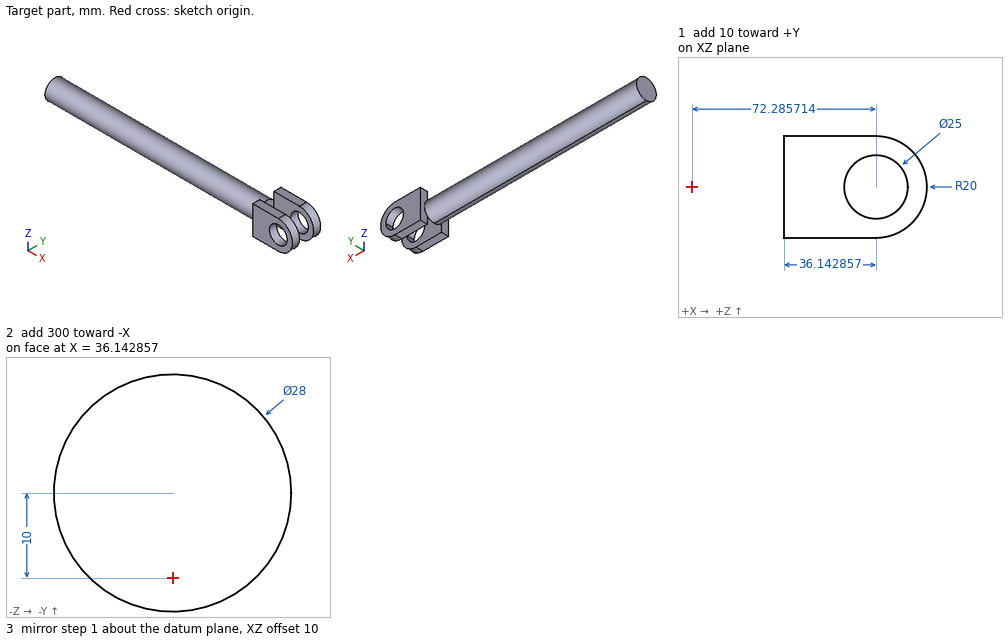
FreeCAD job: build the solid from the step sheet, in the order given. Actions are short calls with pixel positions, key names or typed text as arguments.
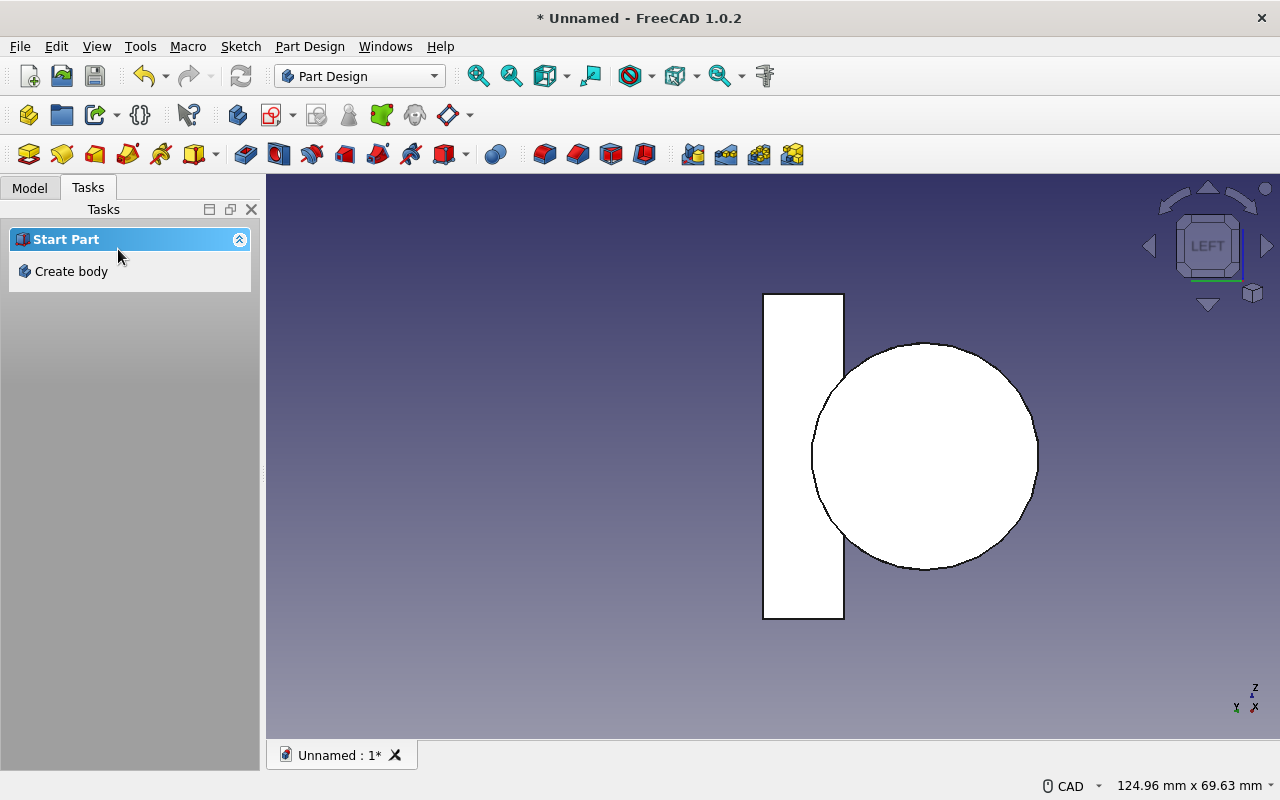
click(30, 188)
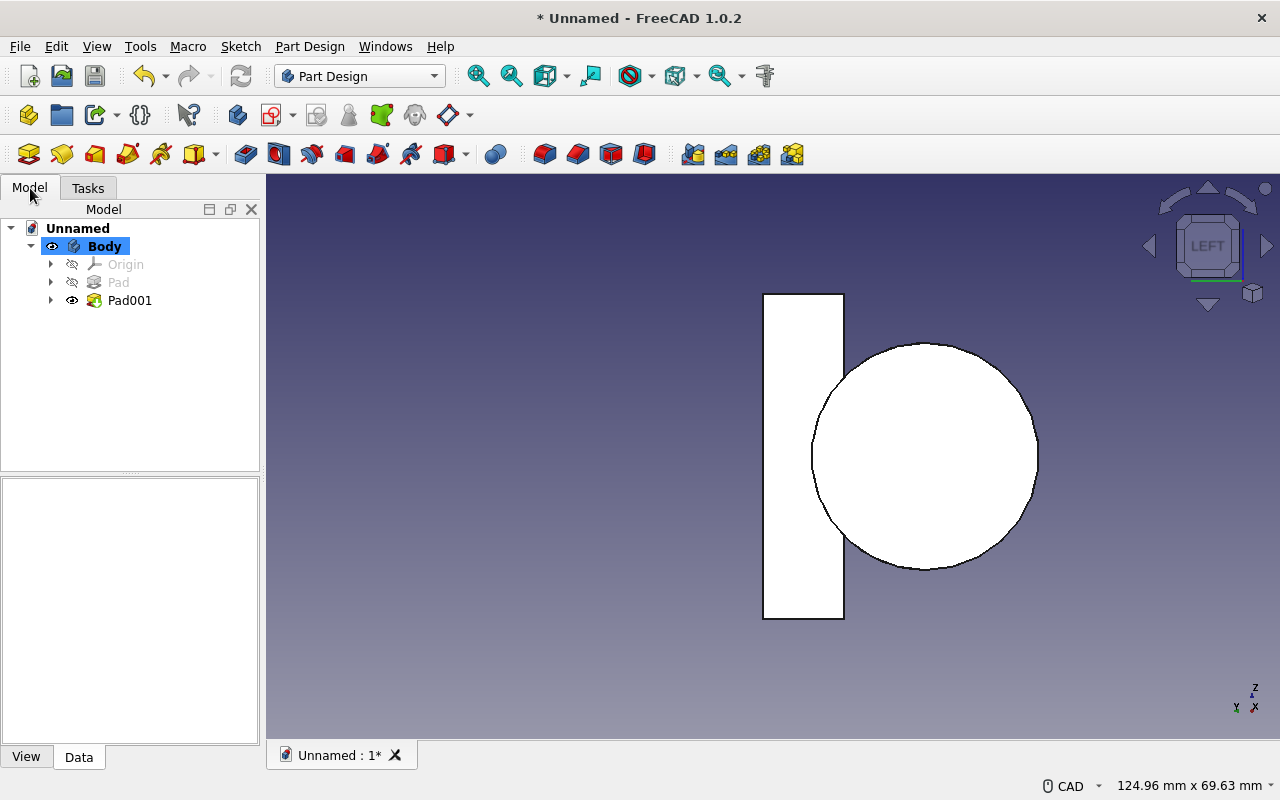
click(51, 264)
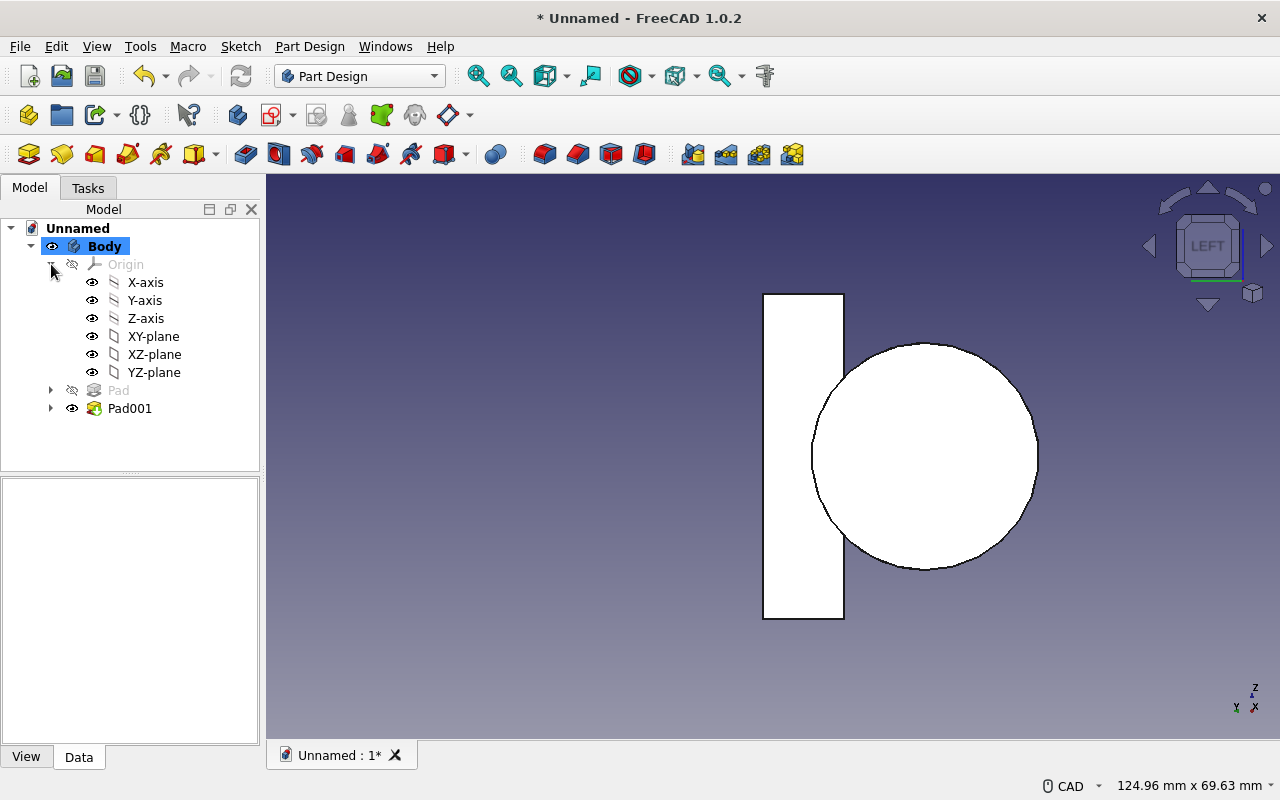
click(137, 354)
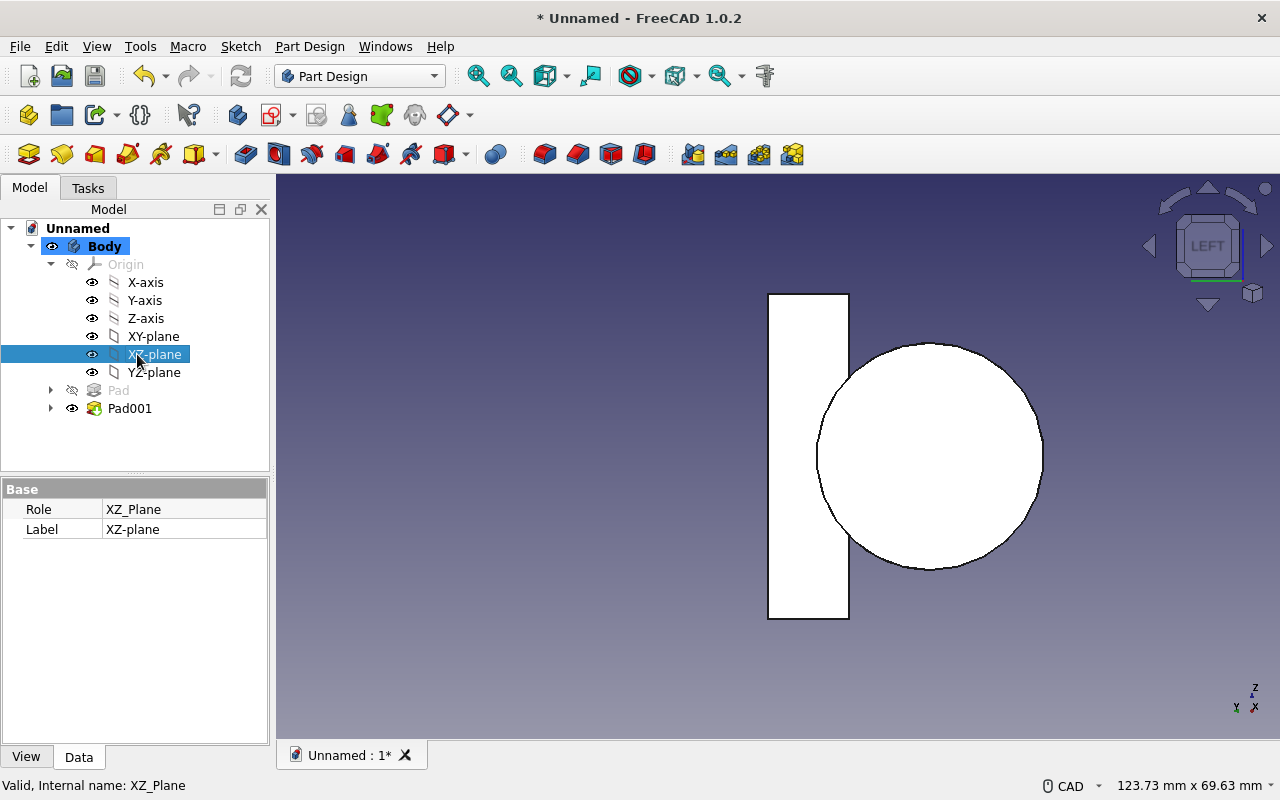
click(448, 116)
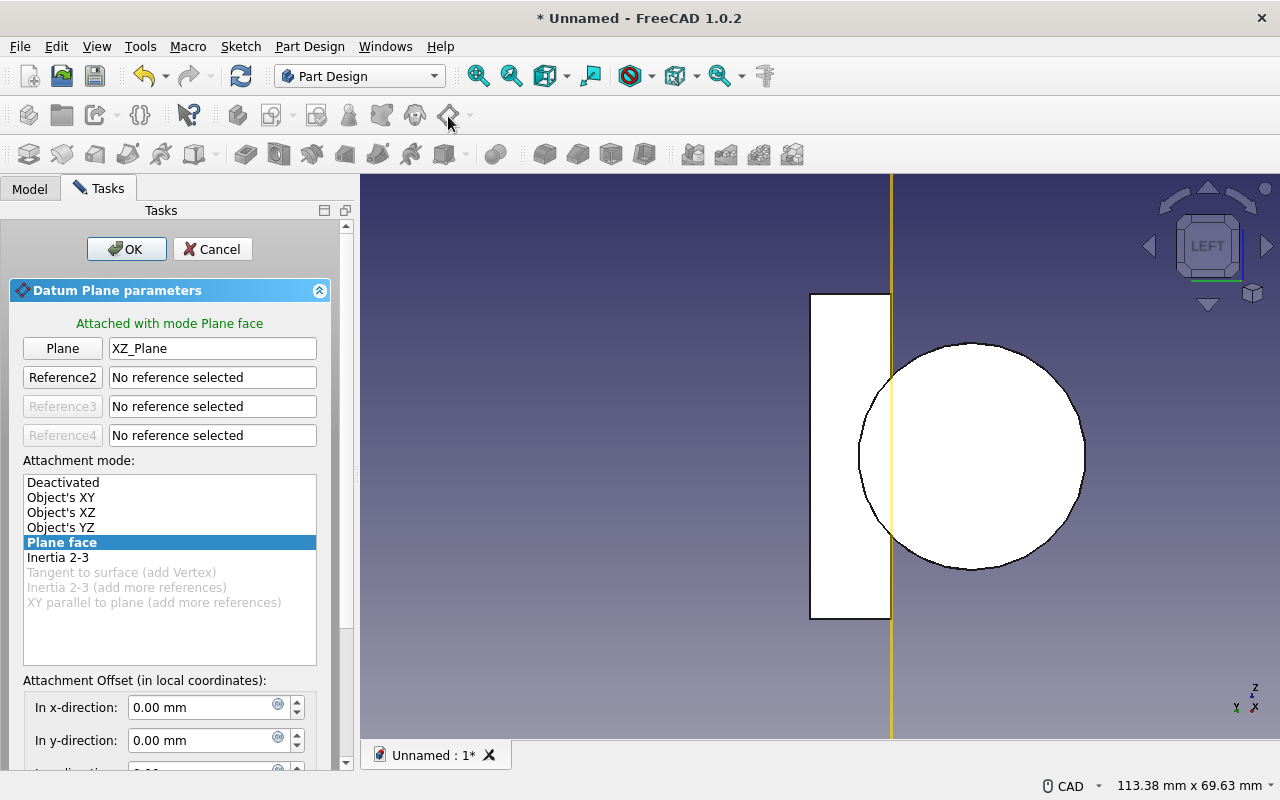
scroll(346, 495, down, 2)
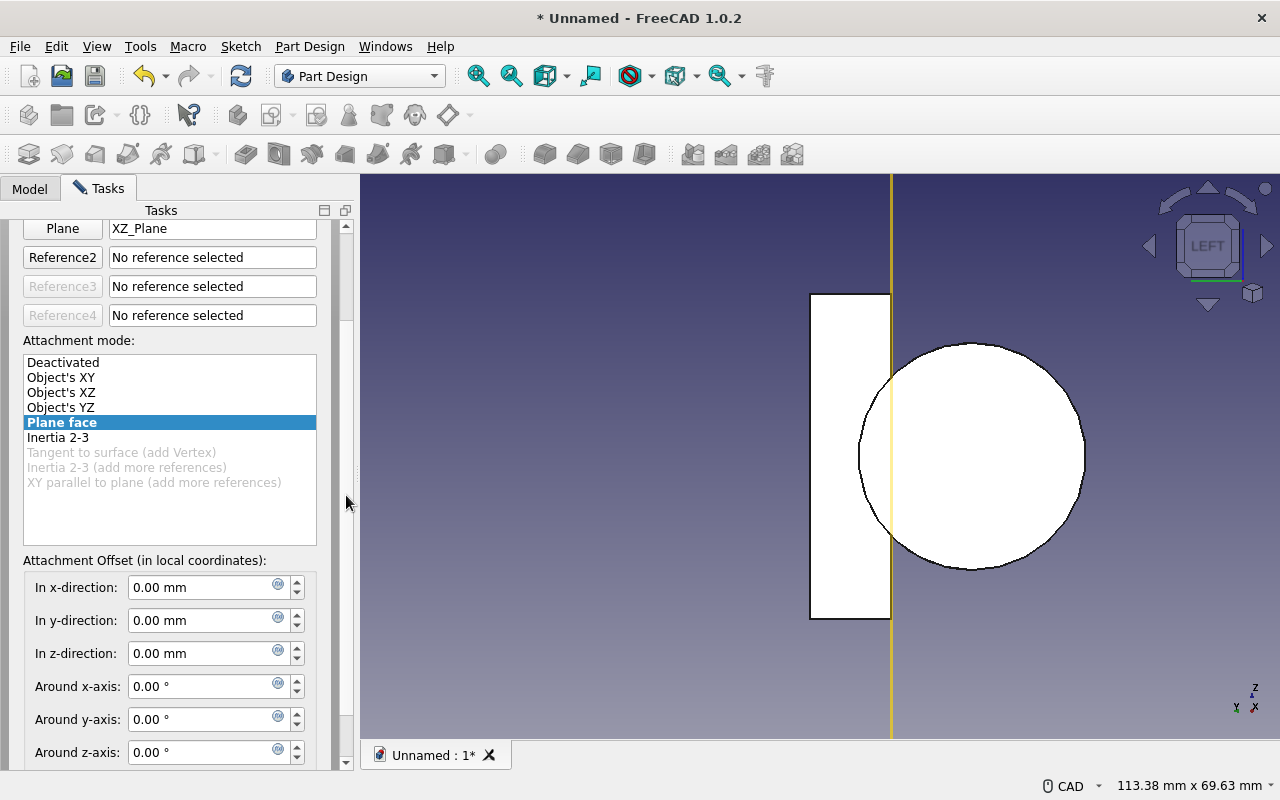
triple_click(210, 654)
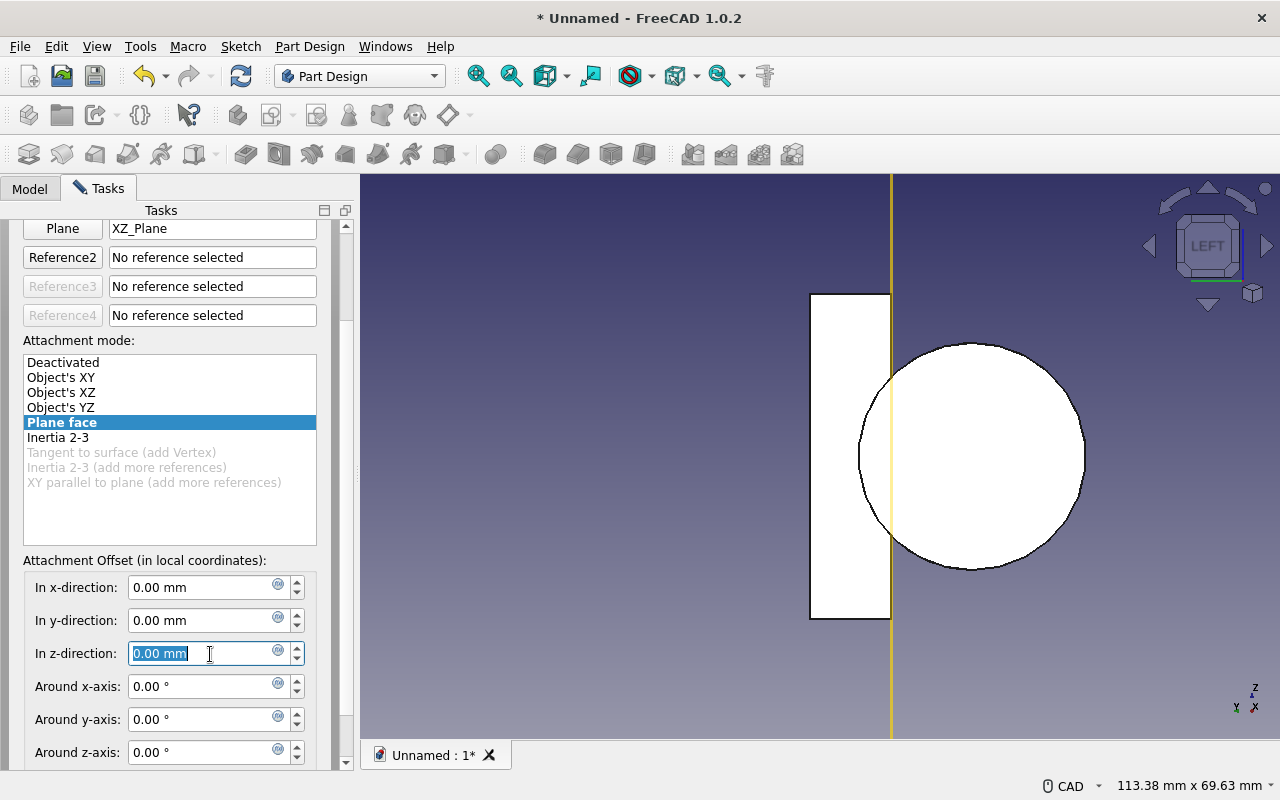
text(10)
key(Tab)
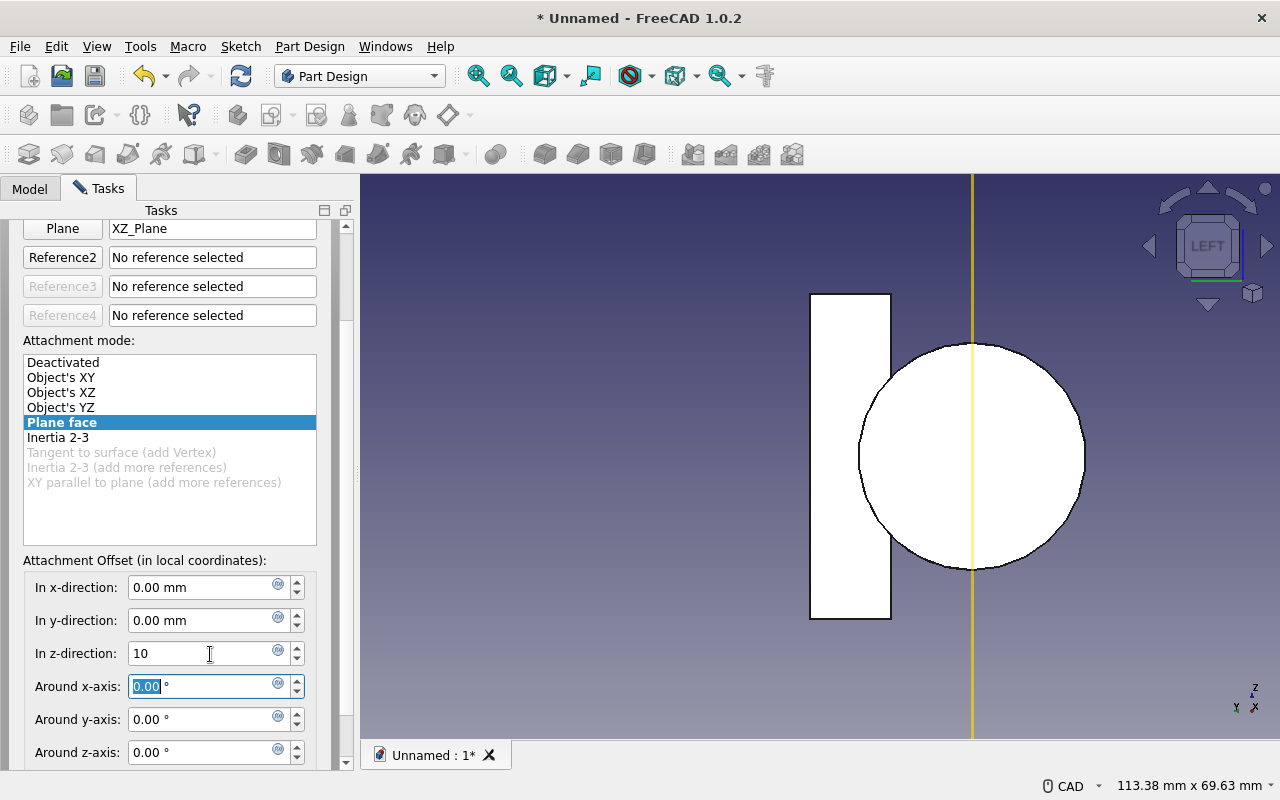
scroll(346, 495, up, 3)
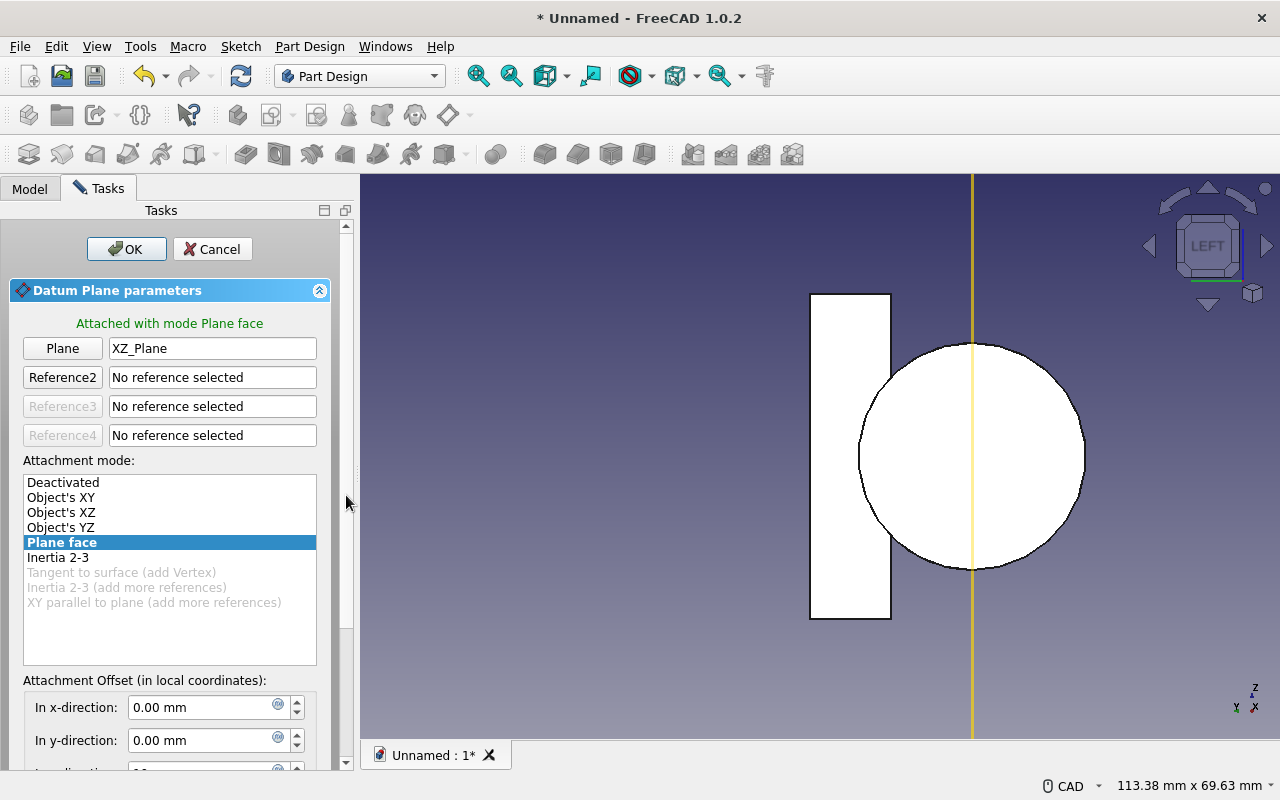
click(127, 249)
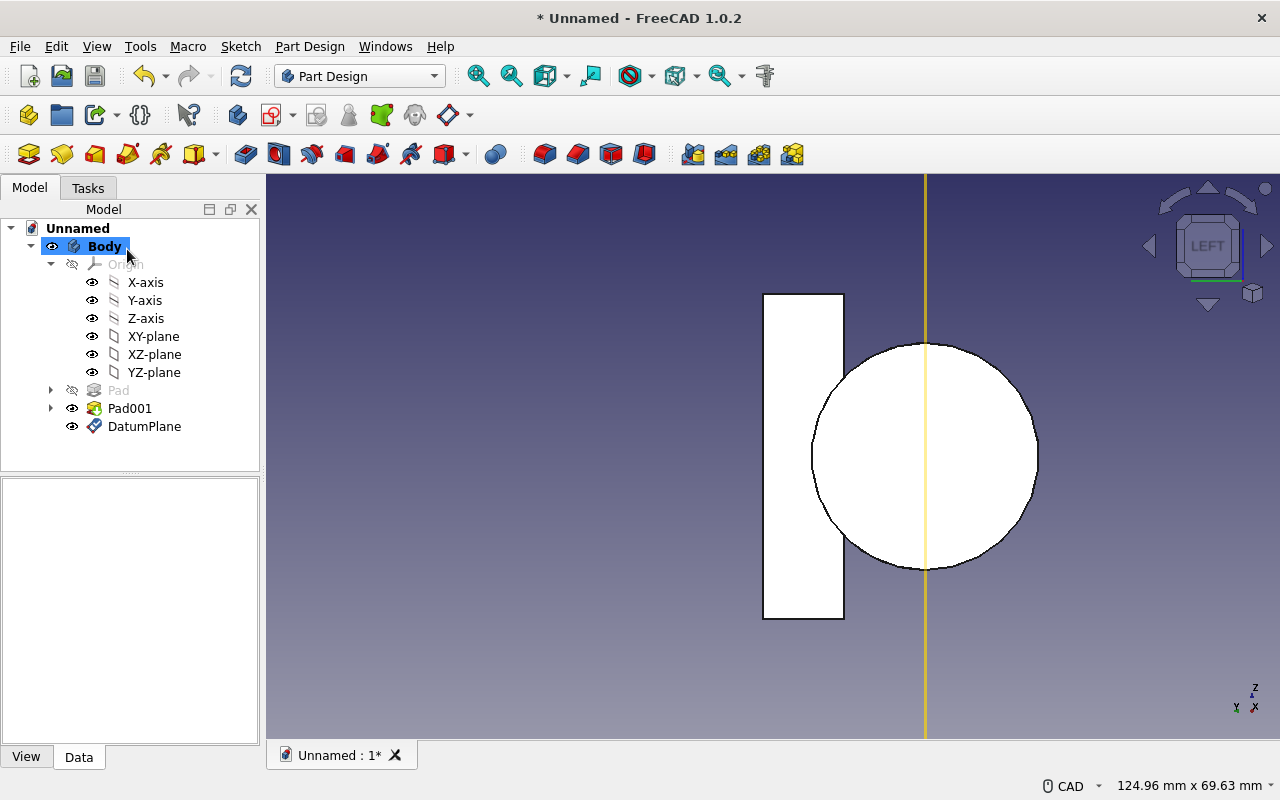
click(117, 390)